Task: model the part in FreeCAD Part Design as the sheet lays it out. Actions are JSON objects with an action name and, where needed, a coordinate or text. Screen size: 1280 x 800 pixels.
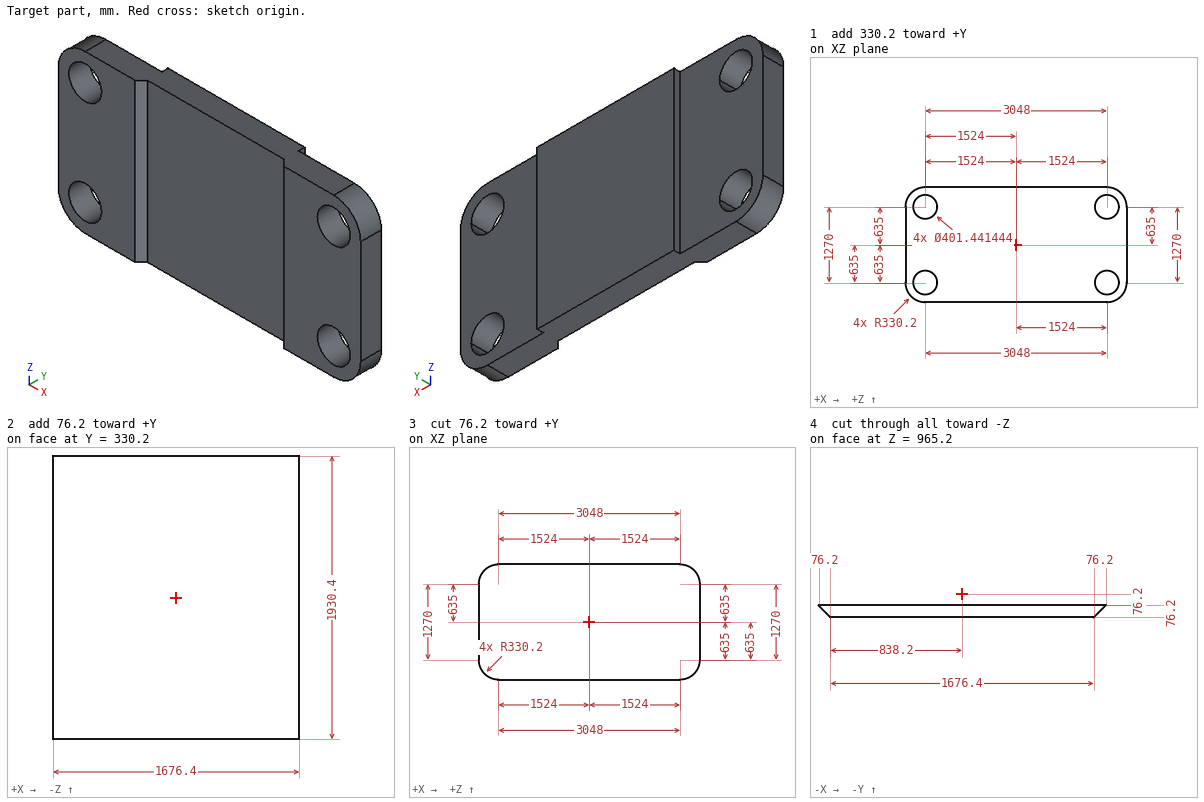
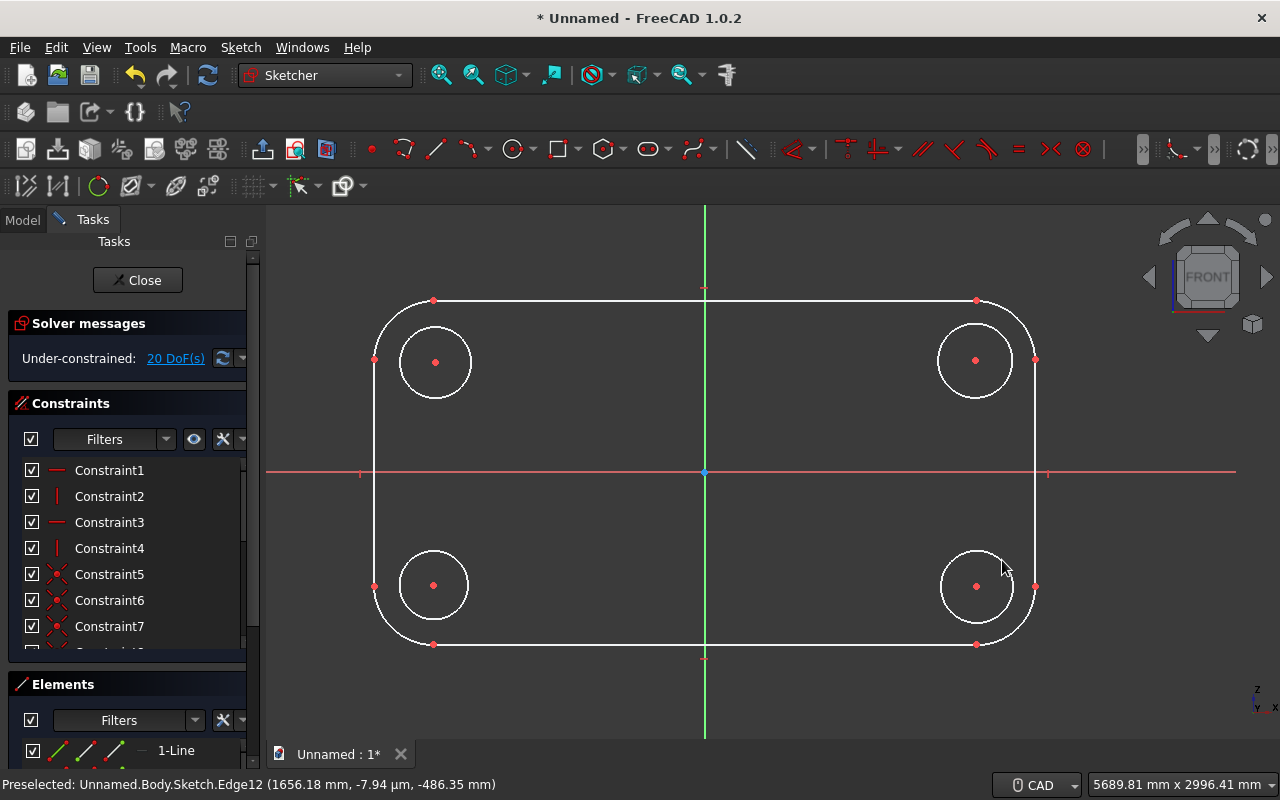
{"action": "left_click", "coordinate": [381, 613]}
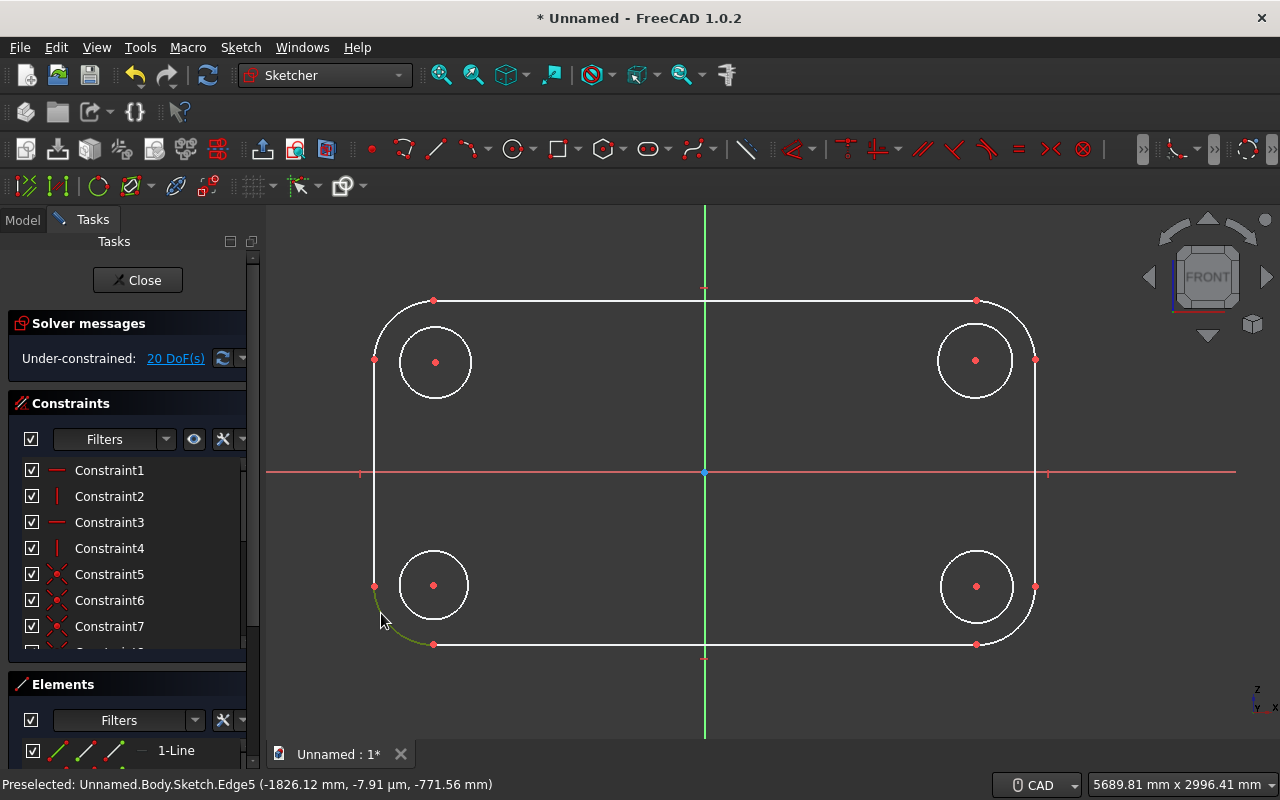
{"action": "left_click", "coordinate": [407, 308]}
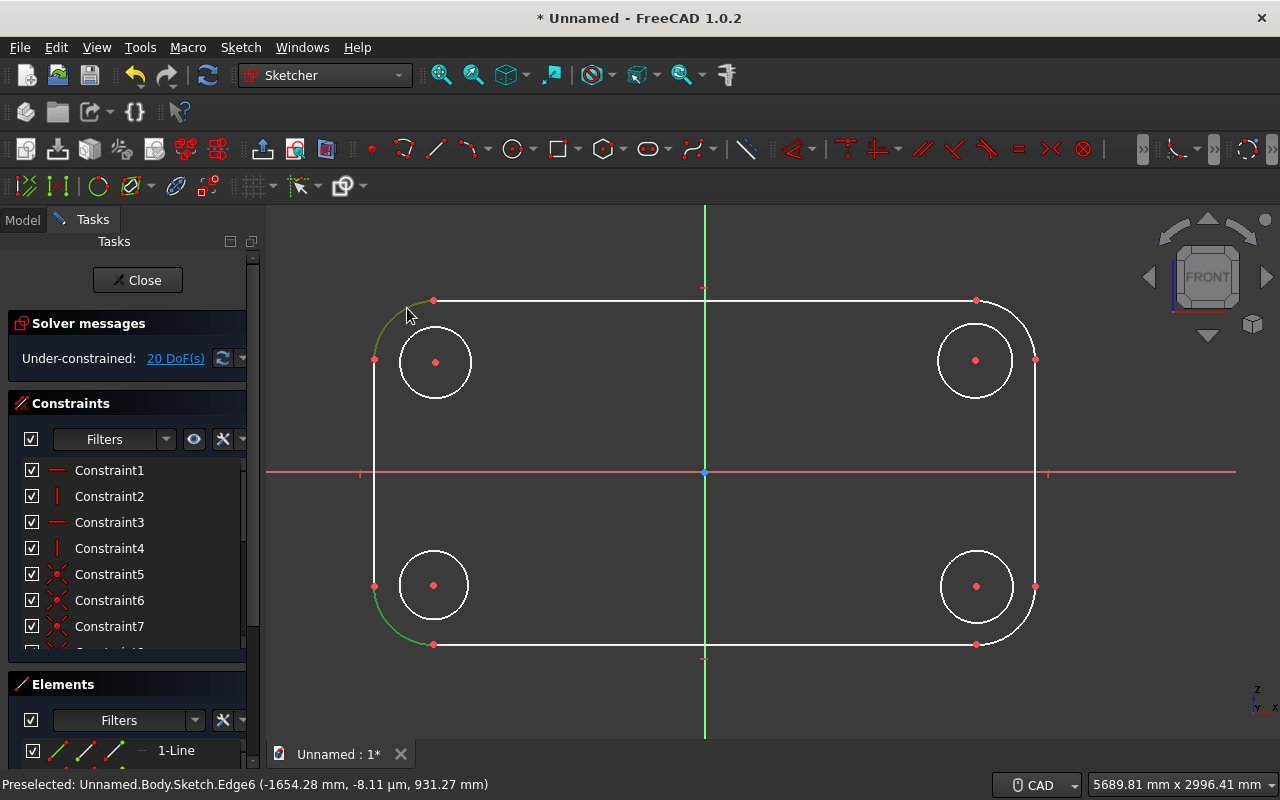
{"action": "left_click", "coordinate": [1028, 333]}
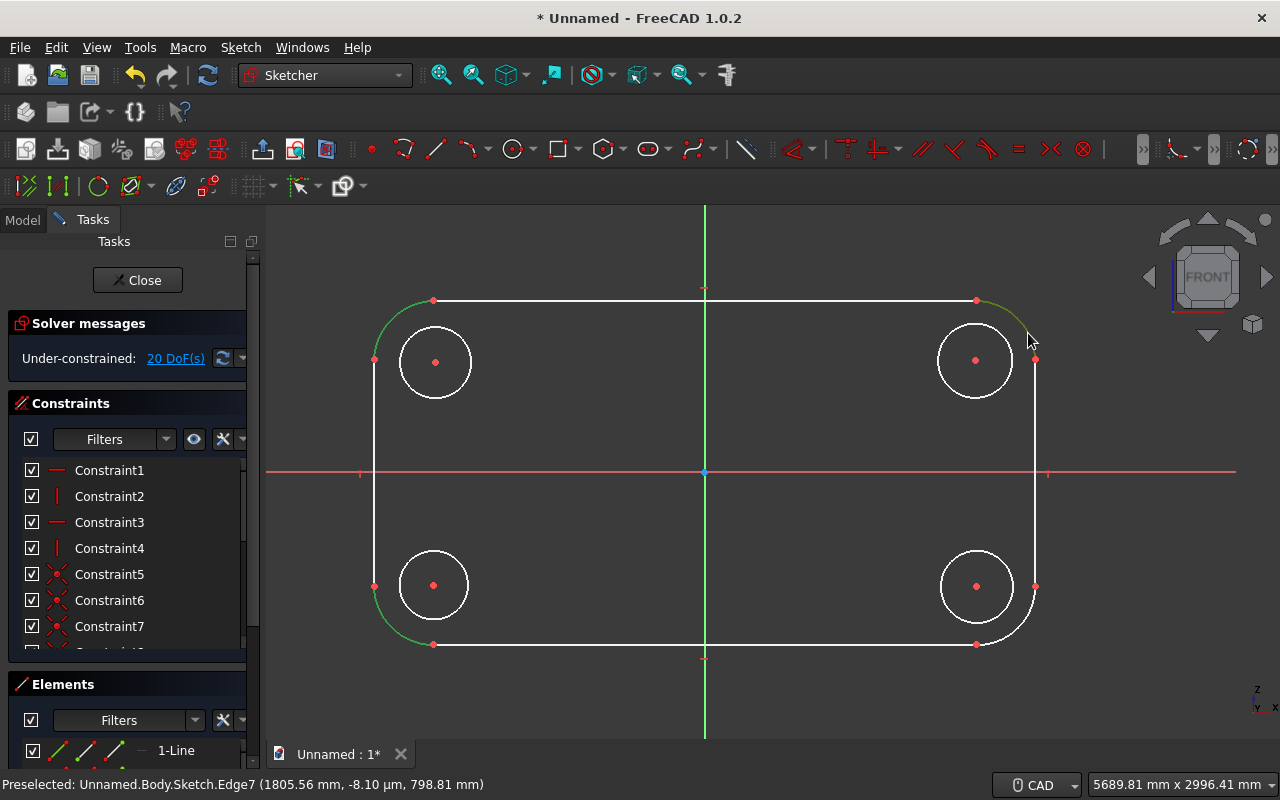
{"action": "left_click", "coordinate": [1003, 639]}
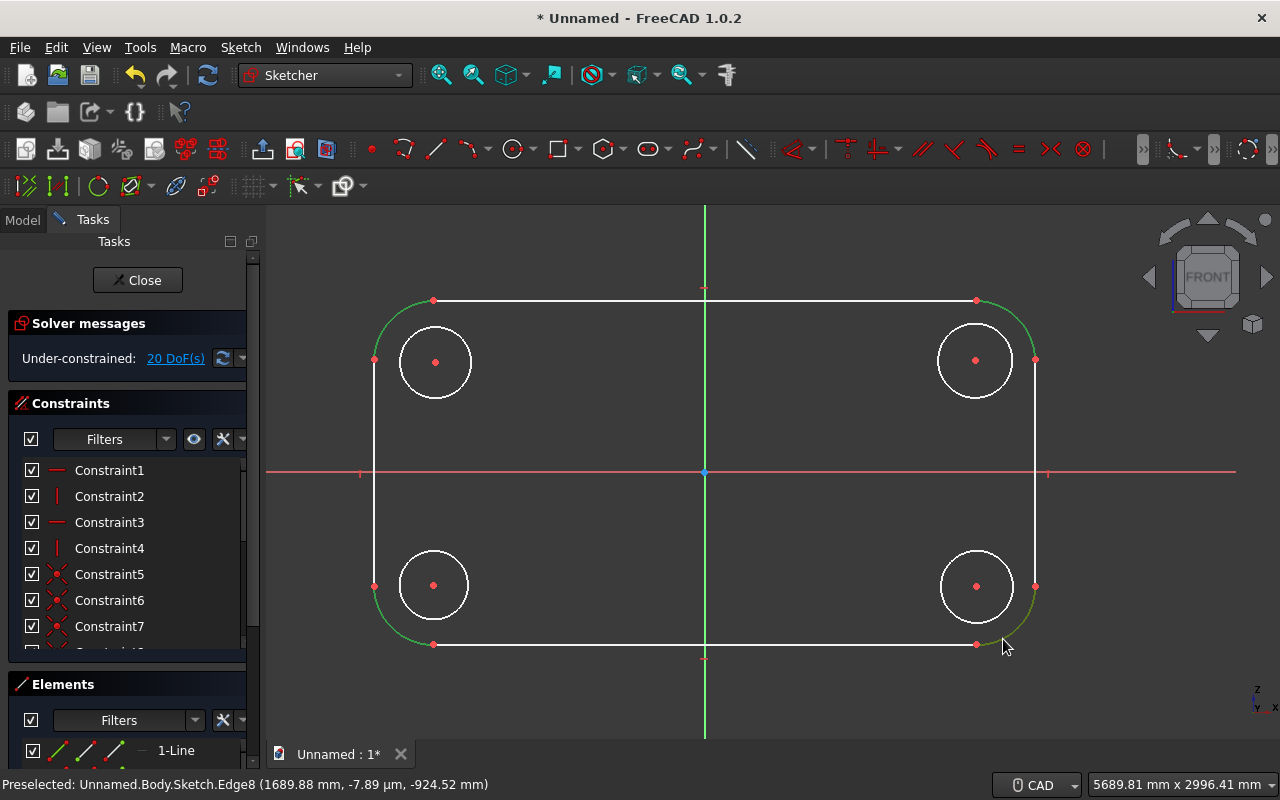
{"action": "key", "text": "e"}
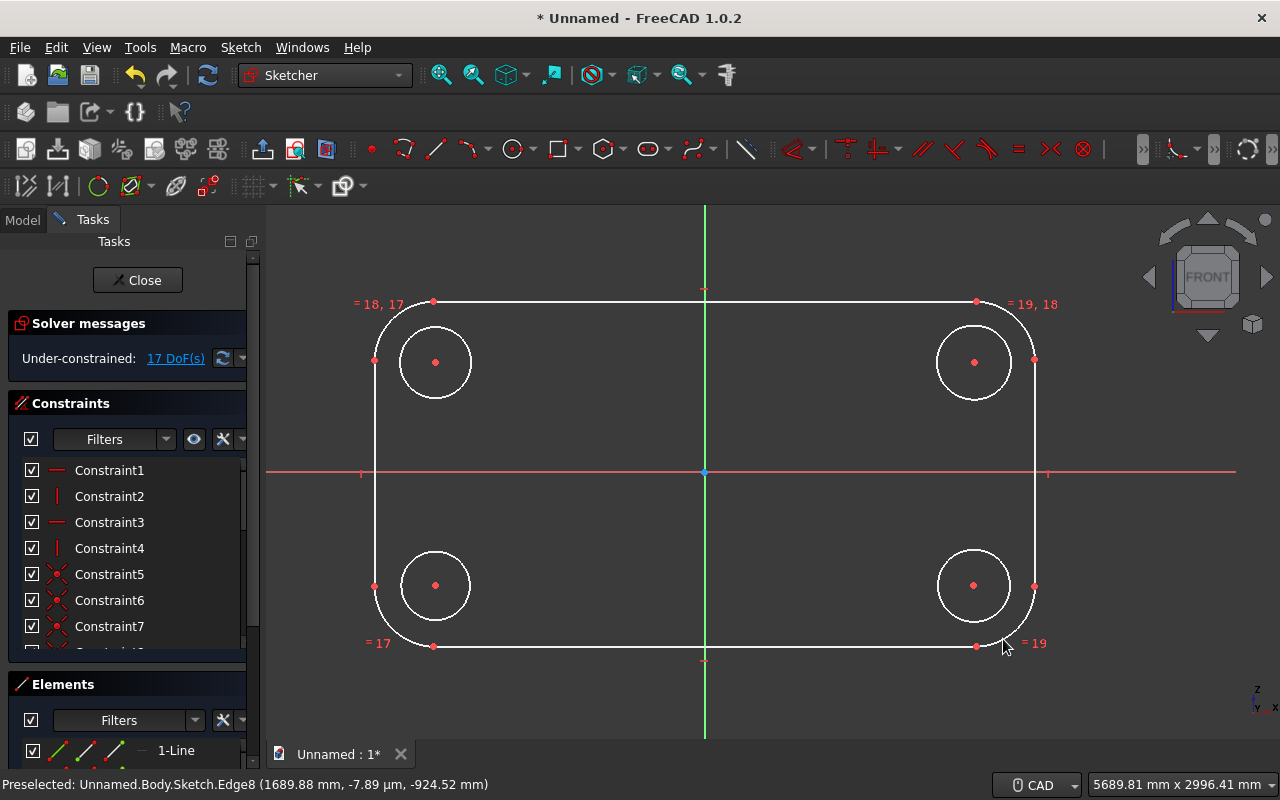
{"action": "left_click", "coordinate": [461, 337]}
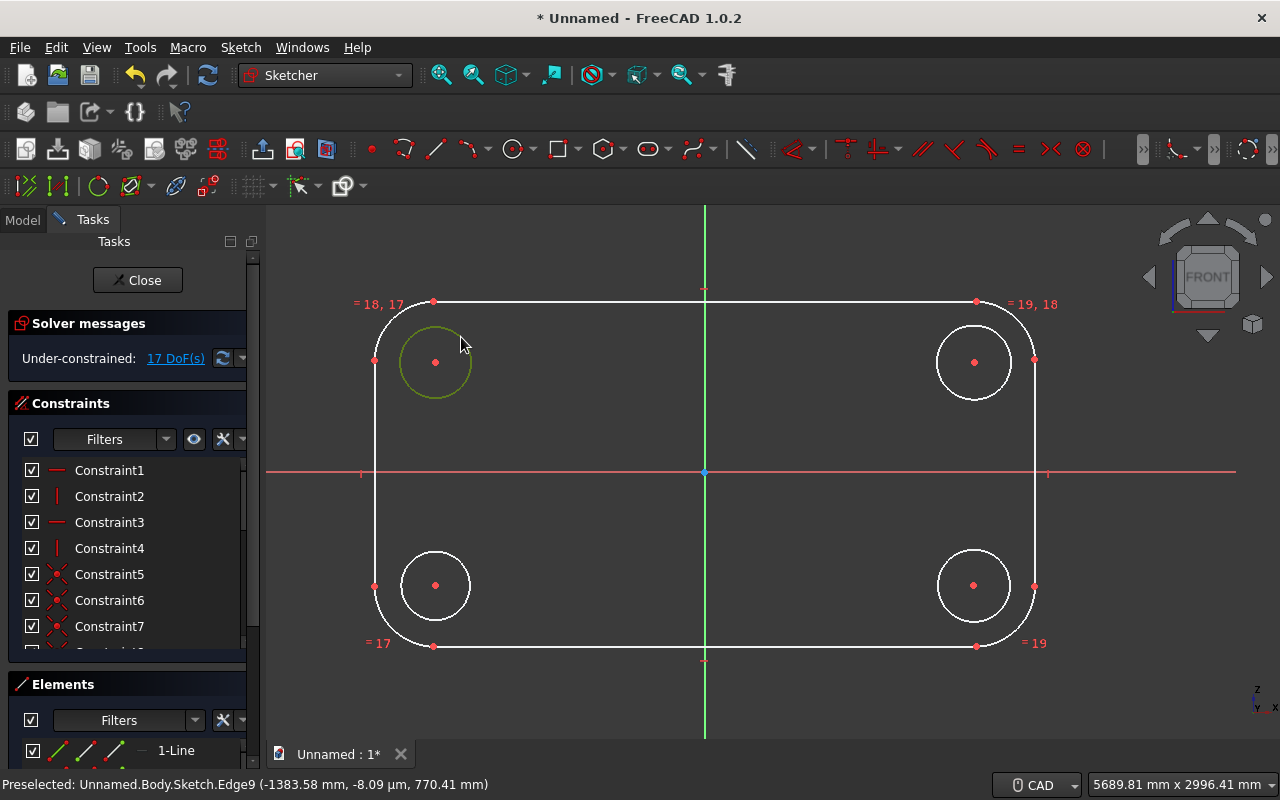
{"action": "left_click", "coordinate": [1000, 336]}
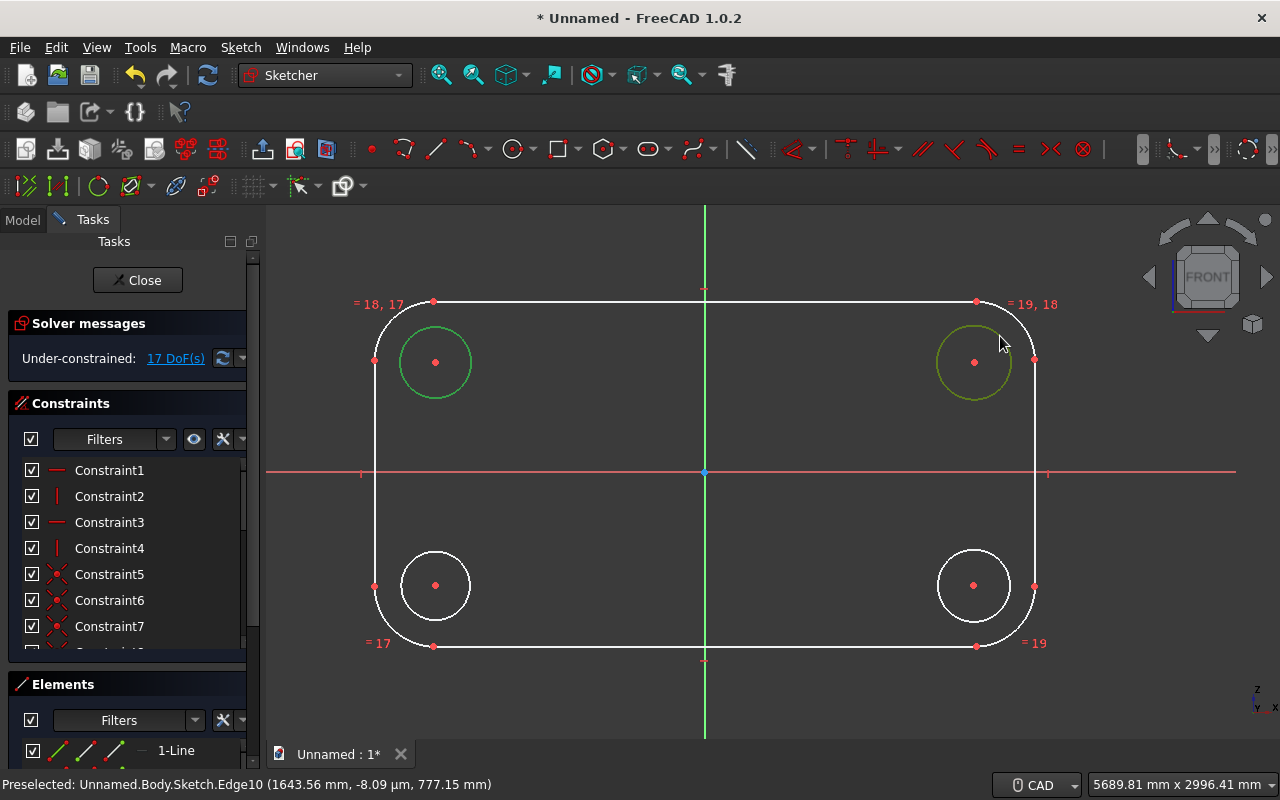
{"action": "left_click", "coordinate": [460, 562]}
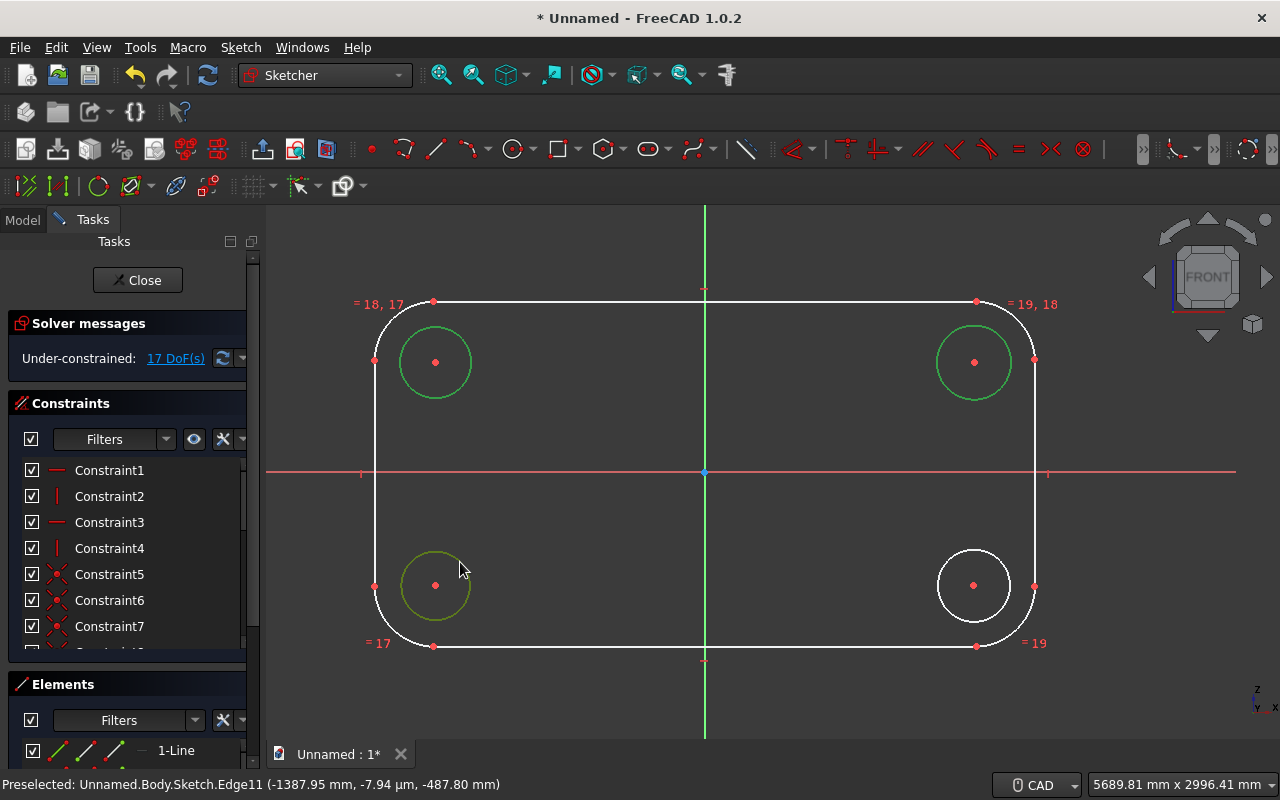
{"action": "left_click", "coordinate": [999, 560]}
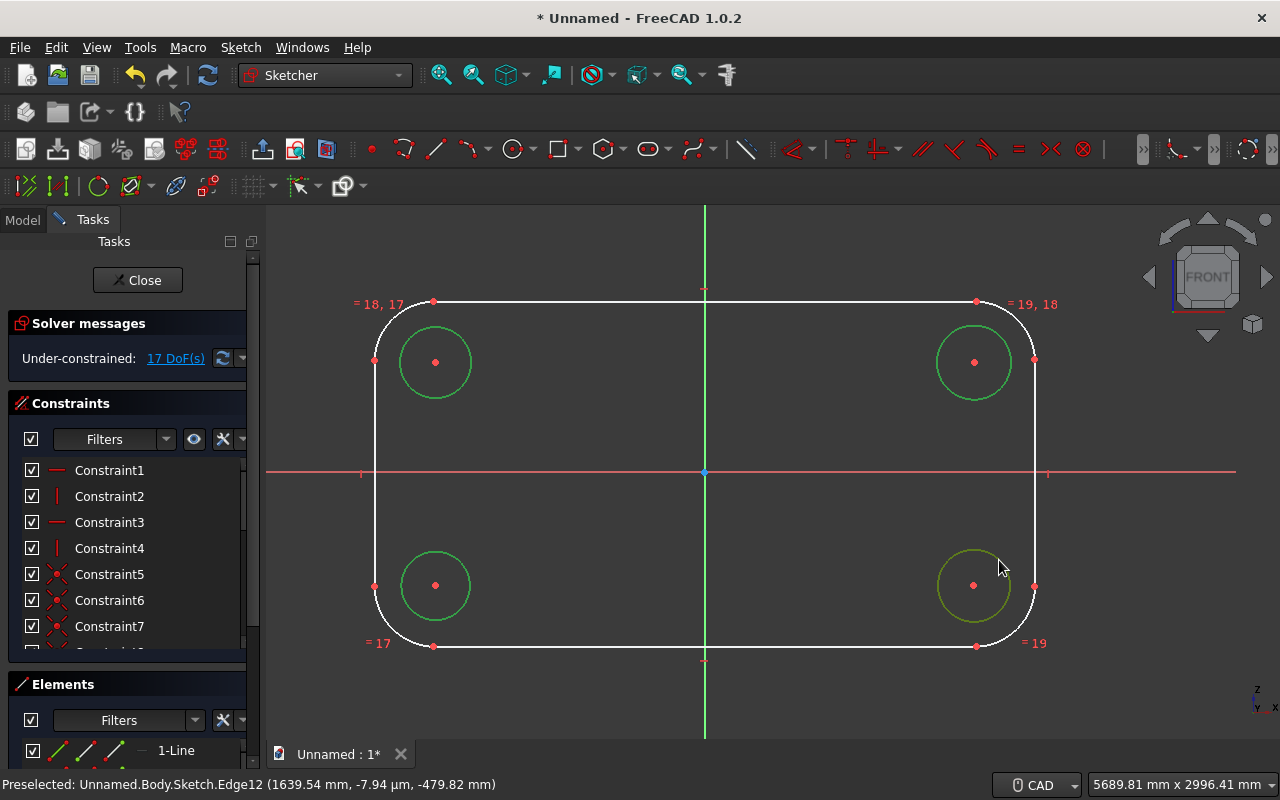
{"action": "key", "text": "e"}